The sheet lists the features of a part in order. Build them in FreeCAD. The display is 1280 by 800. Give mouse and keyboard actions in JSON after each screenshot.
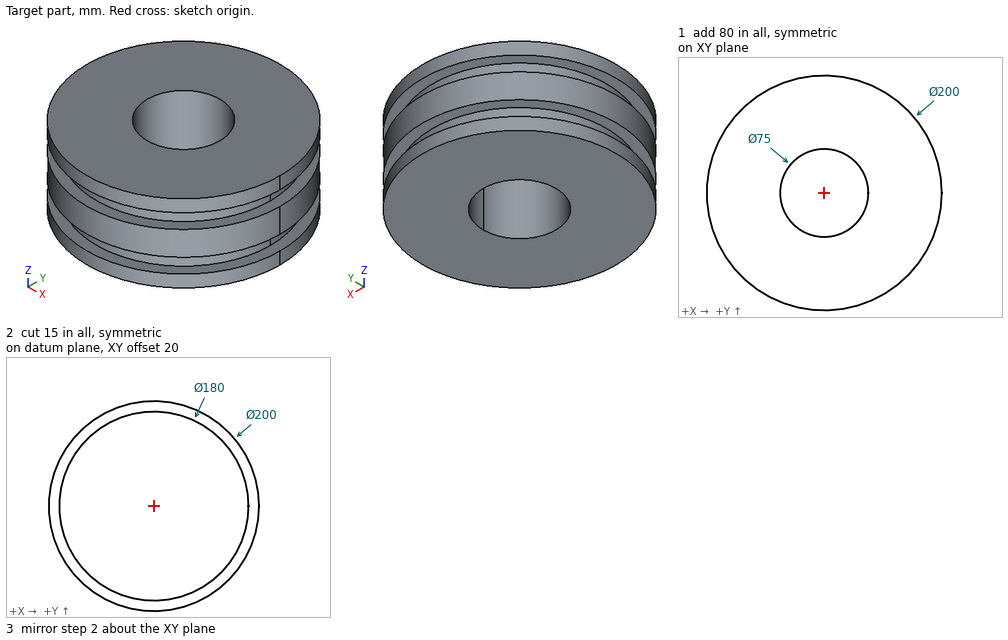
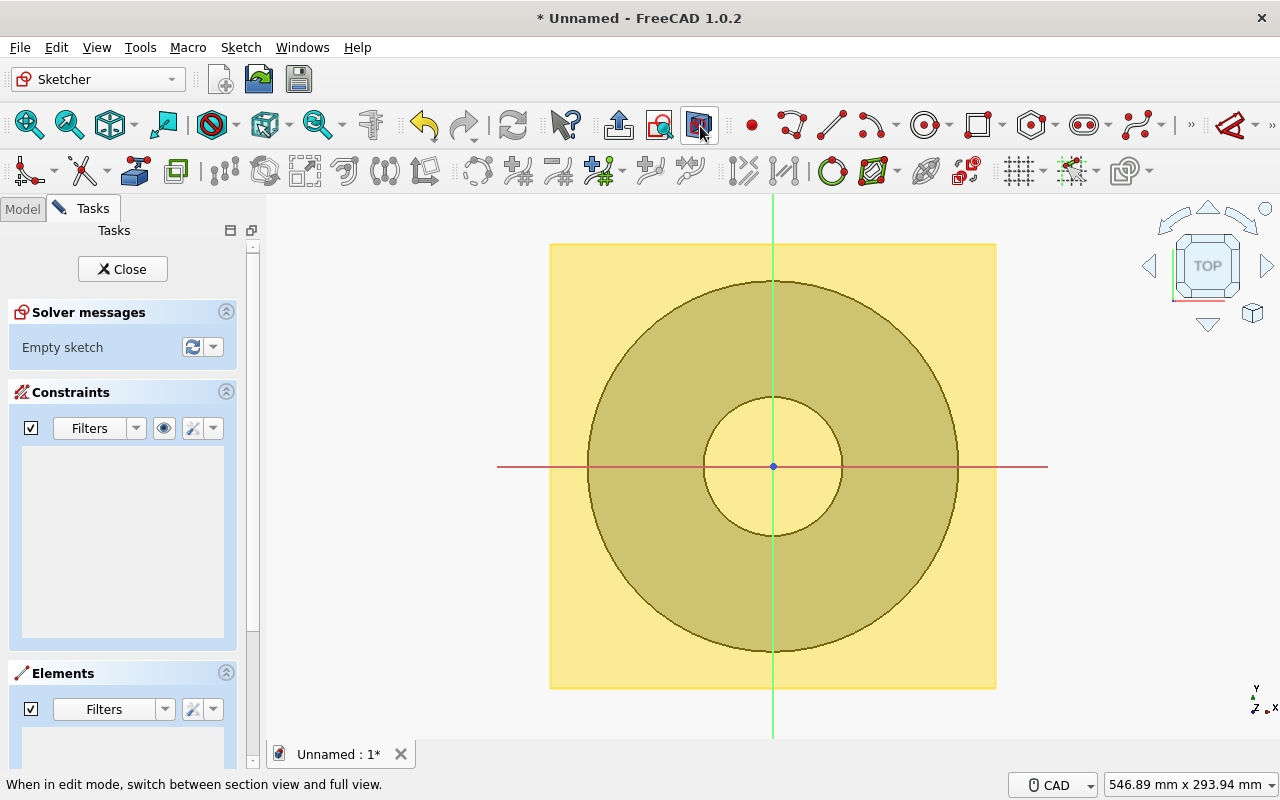
{"action": "left_click", "coordinate": [926, 126]}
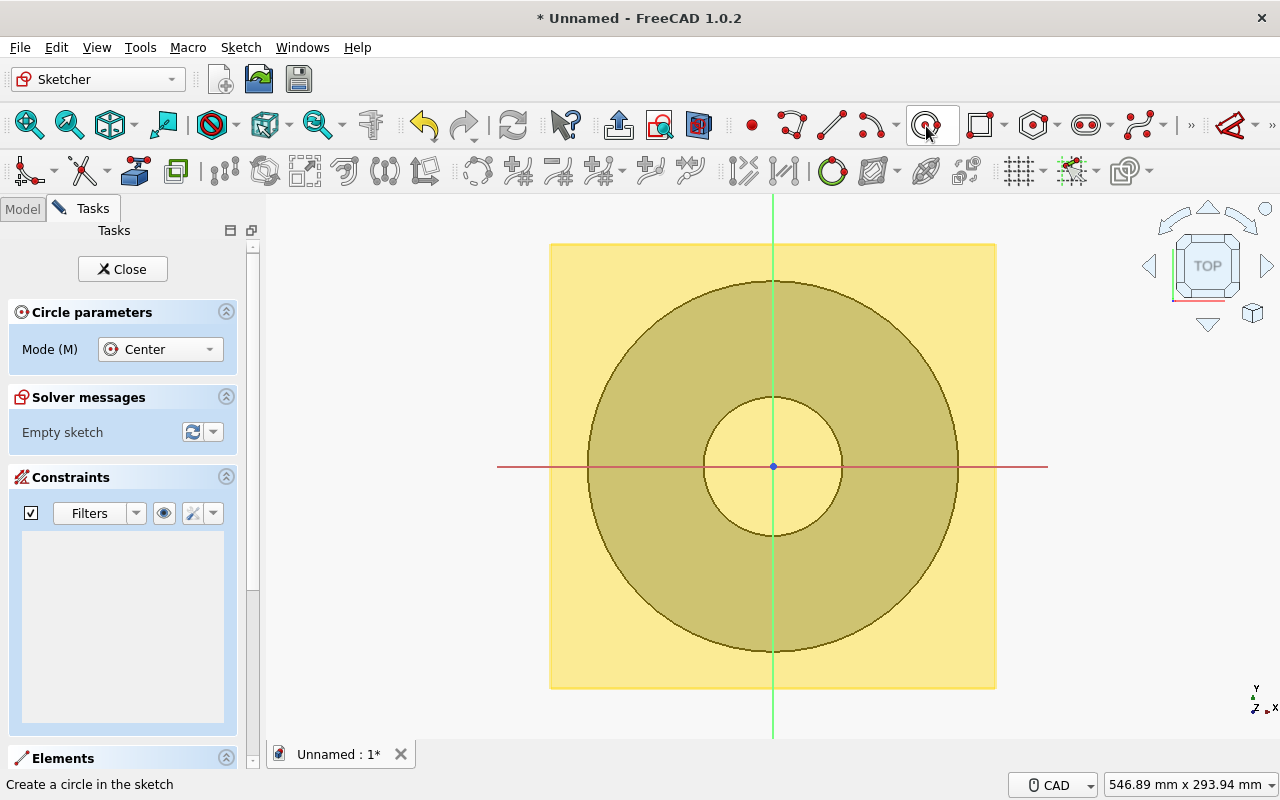
{"action": "left_click", "coordinate": [773, 466]}
{"action": "left_click", "coordinate": [904, 335]}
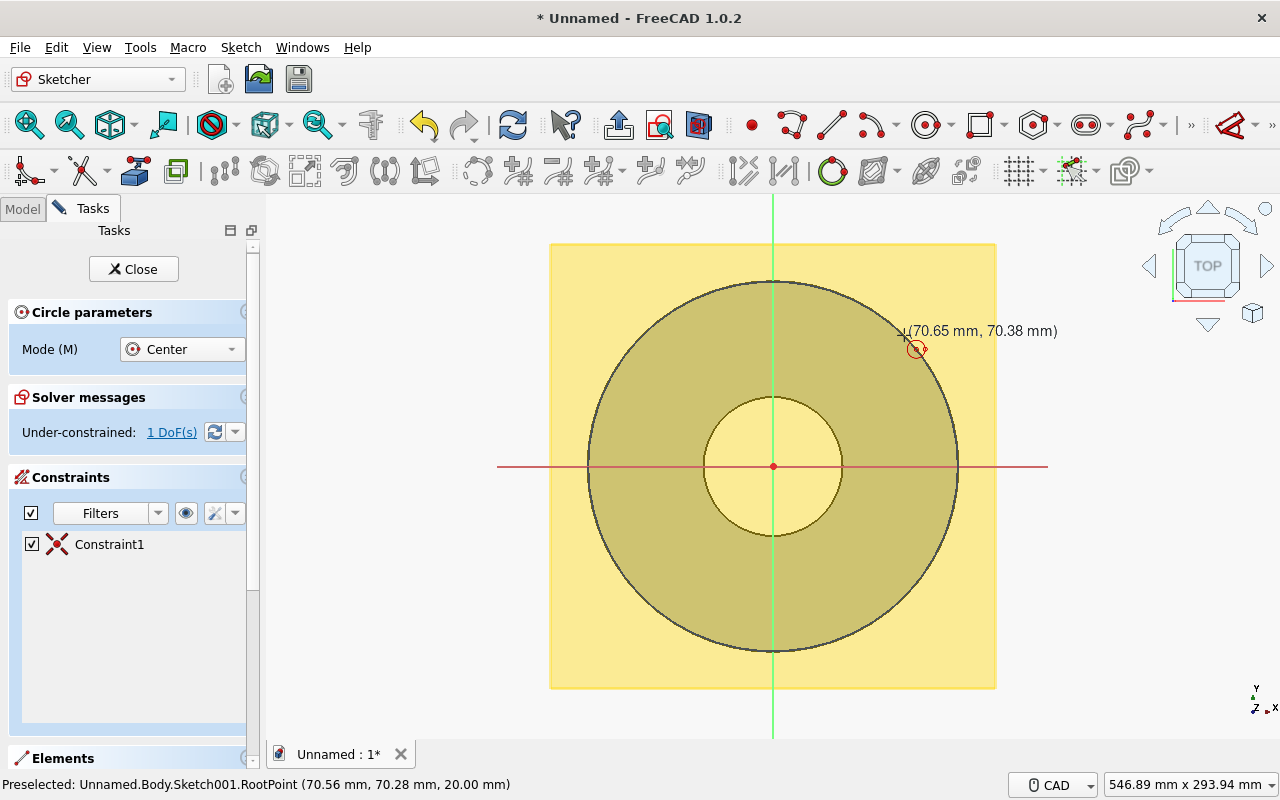
{"action": "left_click", "coordinate": [773, 466]}
{"action": "left_click", "coordinate": [891, 349]}
{"action": "key", "text": "Escape"}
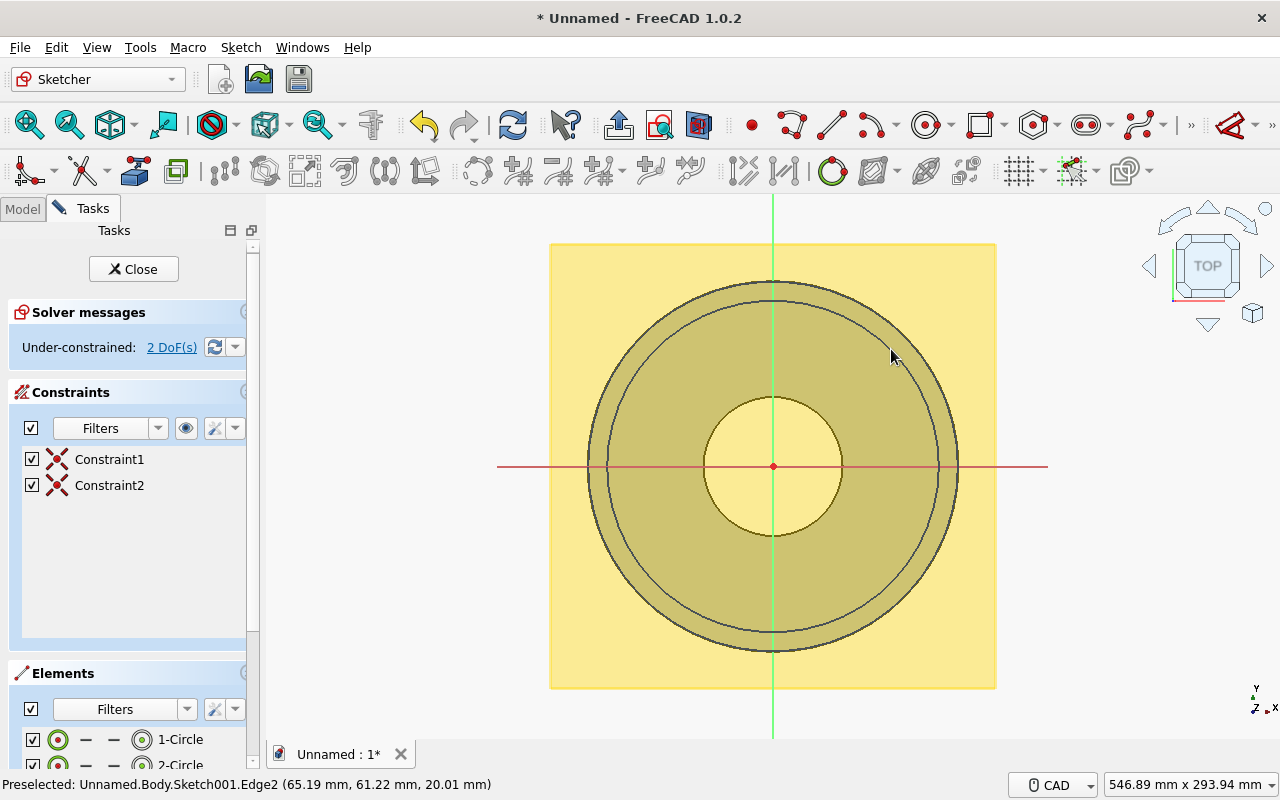
{"action": "left_click", "coordinate": [1230, 126]}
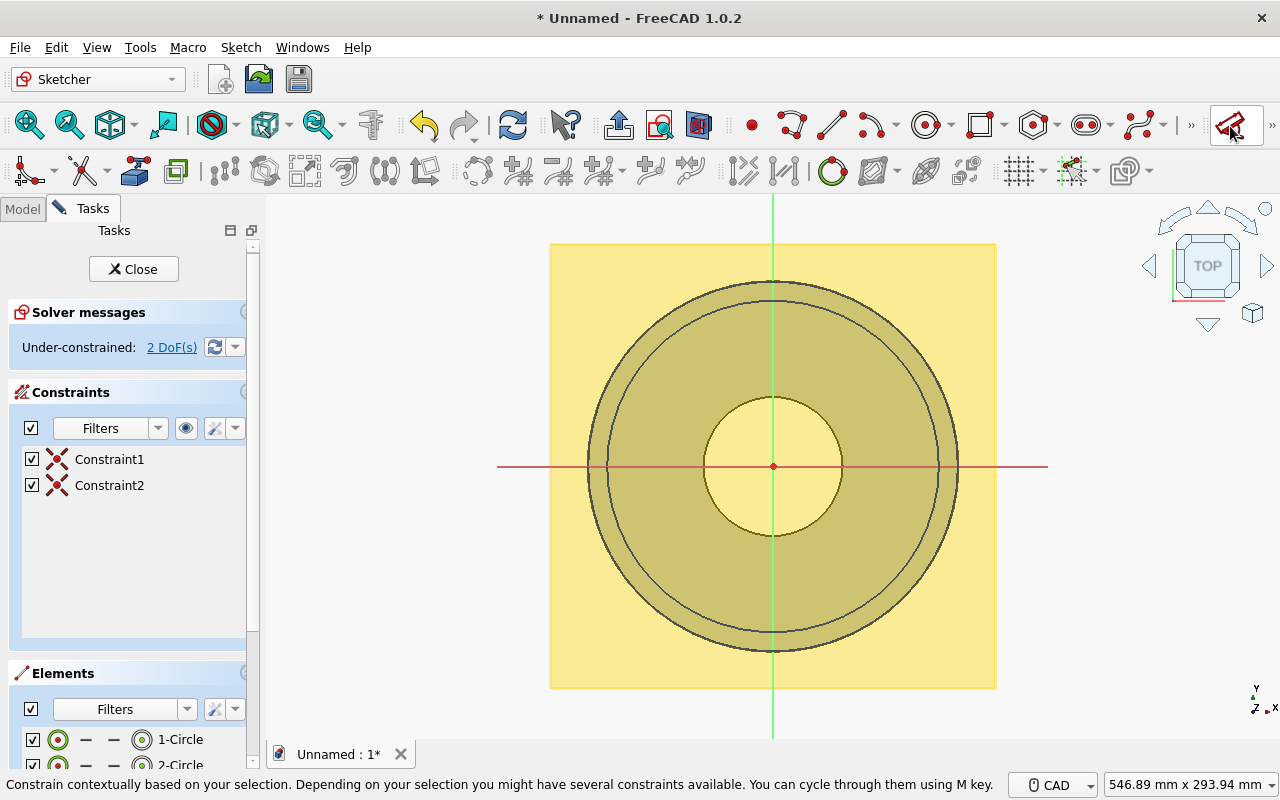
{"action": "left_click", "coordinate": [903, 335]}
{"action": "left_click", "coordinate": [925, 312]}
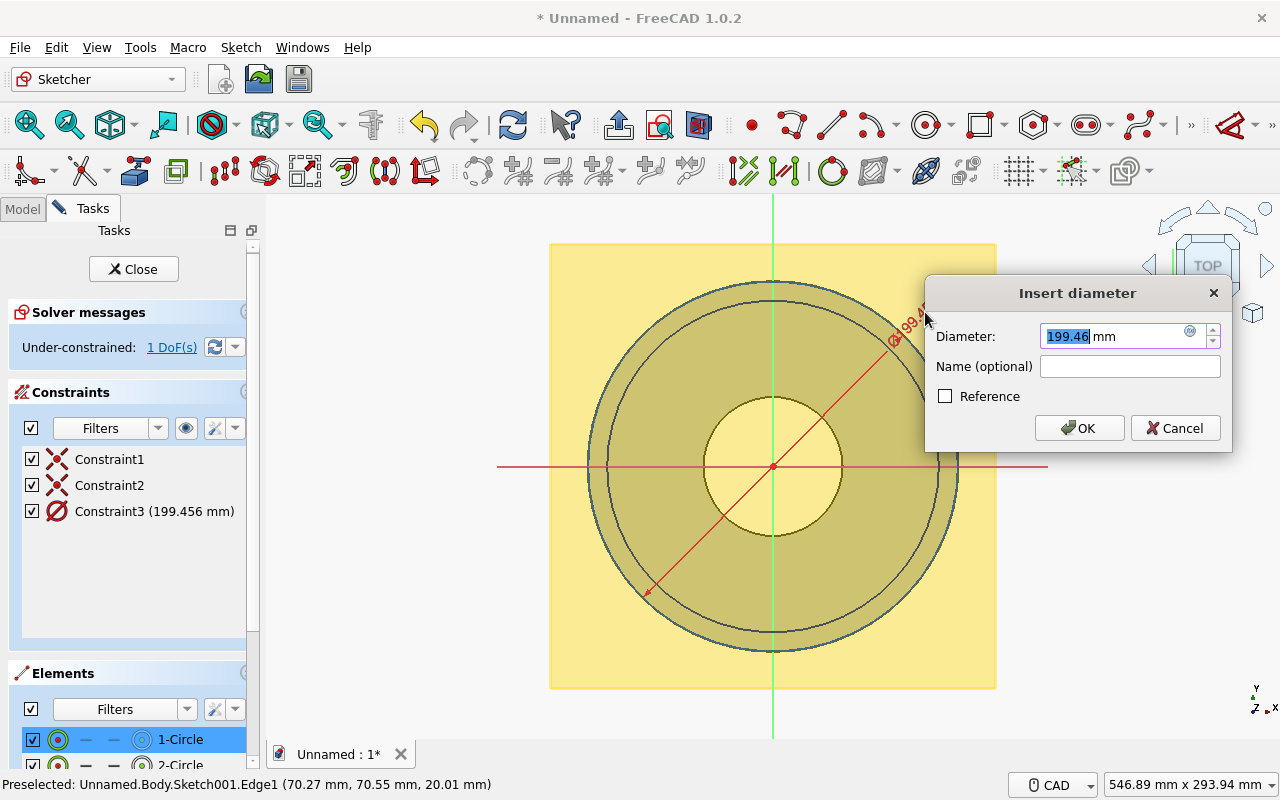
{"action": "type", "text": "200"}
{"action": "key", "text": "Return"}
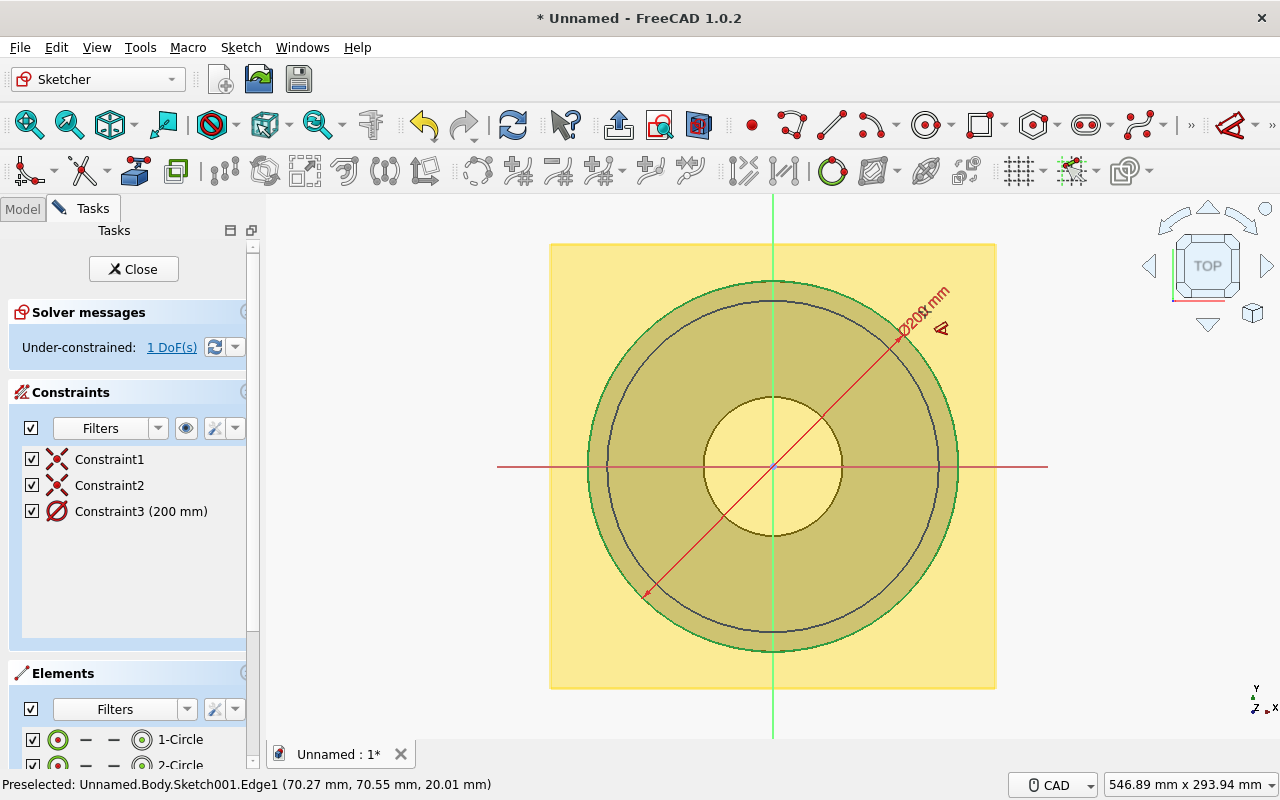
{"action": "left_click", "coordinate": [890, 349]}
{"action": "left_click", "coordinate": [985, 404]}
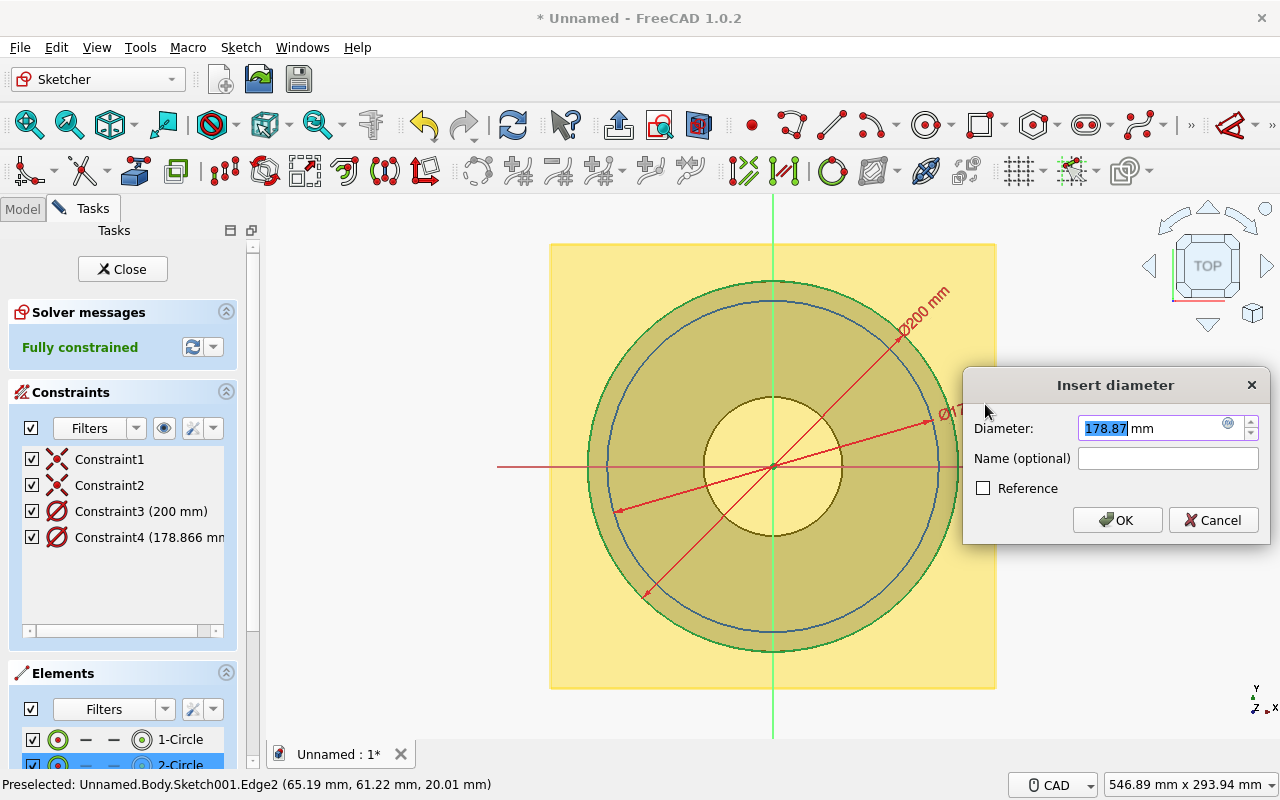
{"action": "type", "text": "180"}
{"action": "key", "text": "Return"}
{"action": "key", "text": "Escape"}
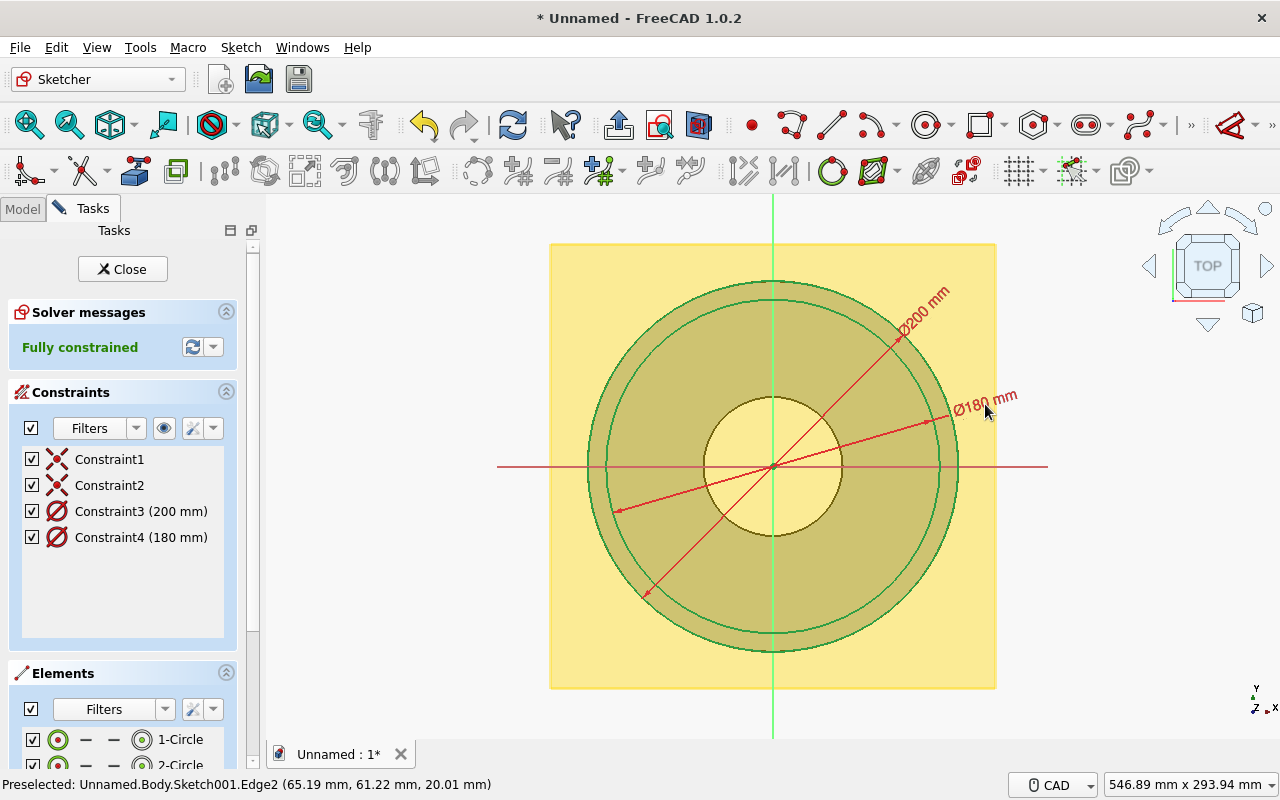
{"action": "left_click", "coordinate": [123, 269]}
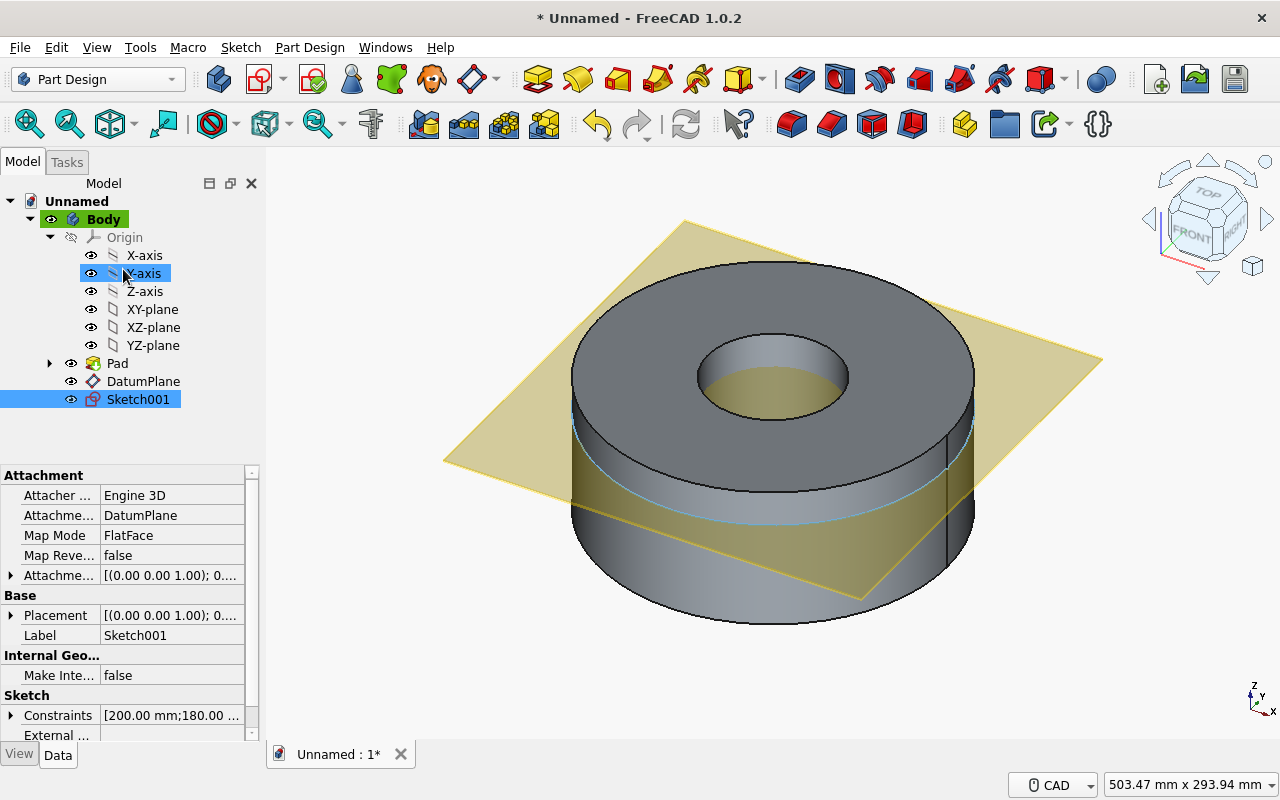
{"action": "left_click", "coordinate": [800, 80]}